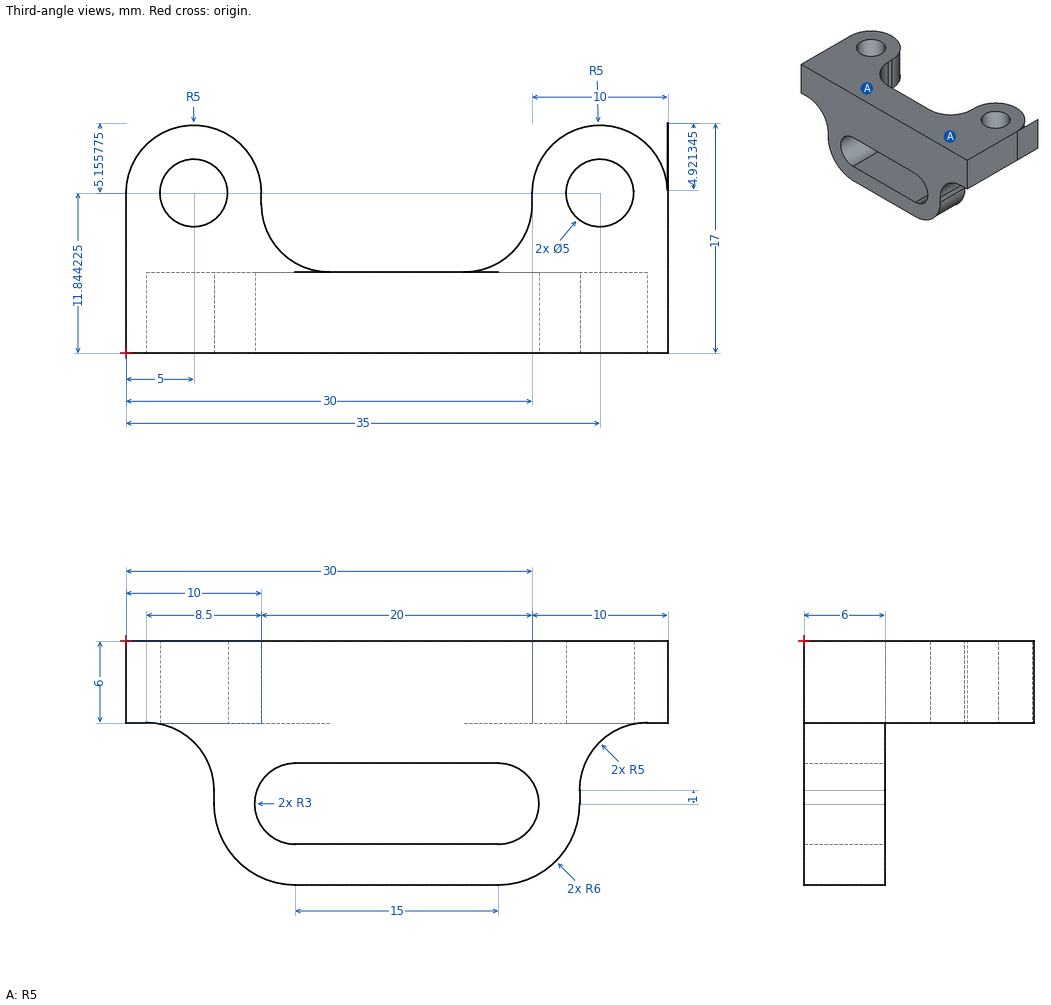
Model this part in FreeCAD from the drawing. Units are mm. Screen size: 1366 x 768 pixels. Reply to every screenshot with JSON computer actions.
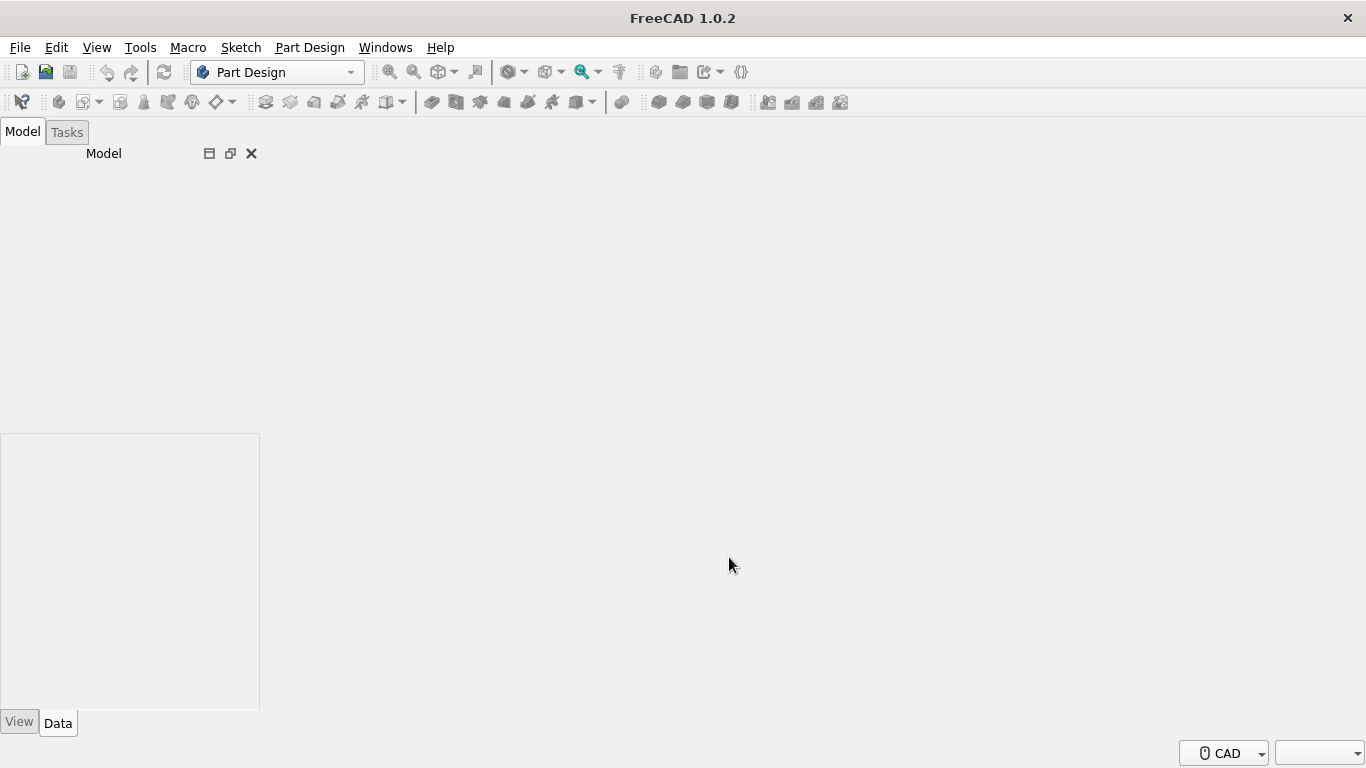
{"action": "key", "text": "ctrl+n"}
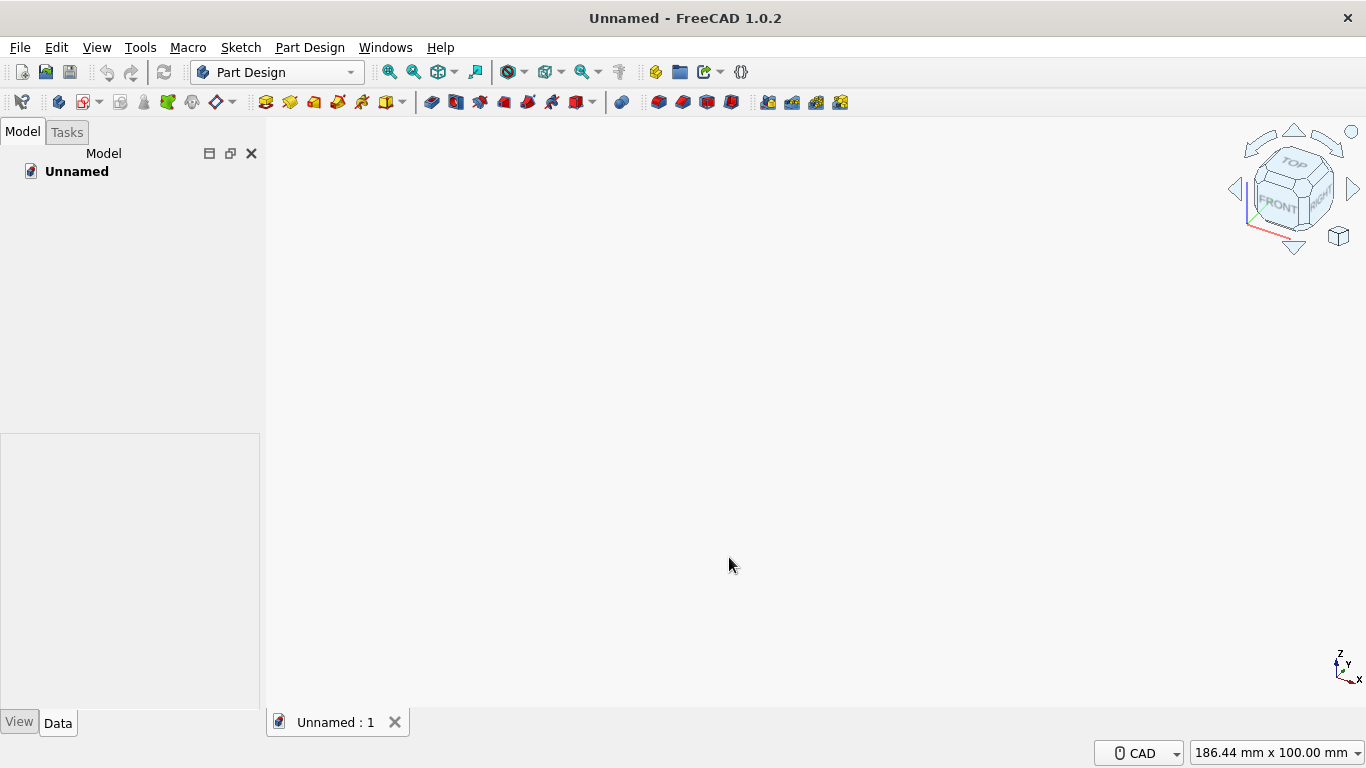
{"action": "left_click", "coordinate": [84, 102]}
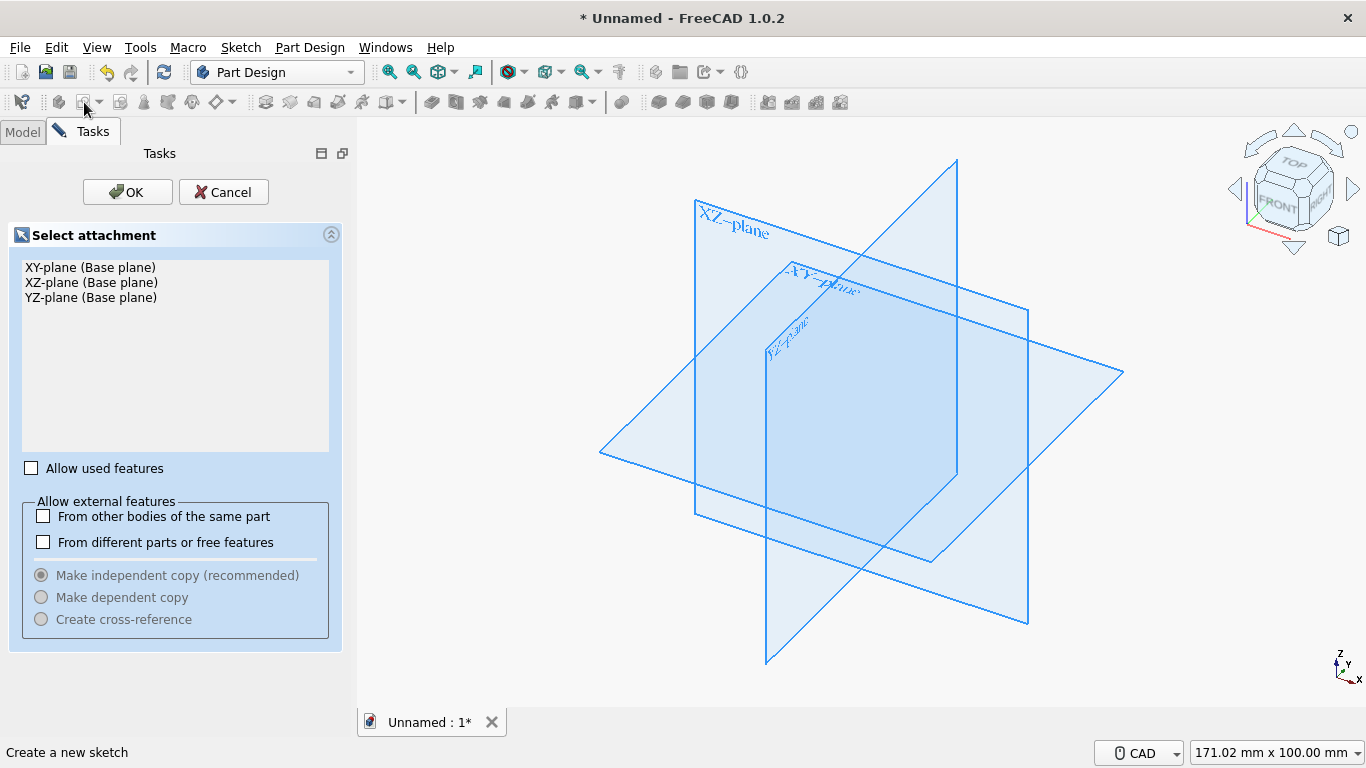
{"action": "left_click", "coordinate": [82, 282]}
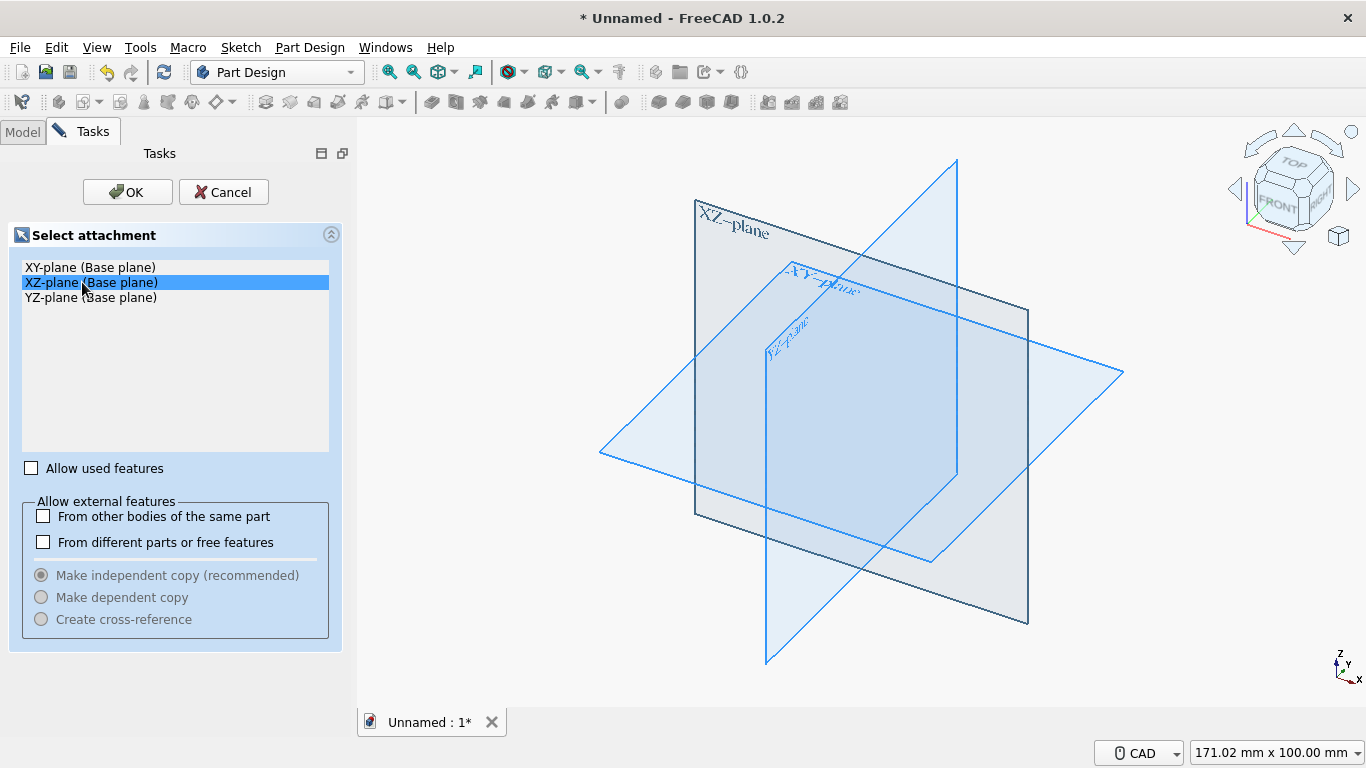
{"action": "left_click", "coordinate": [128, 192]}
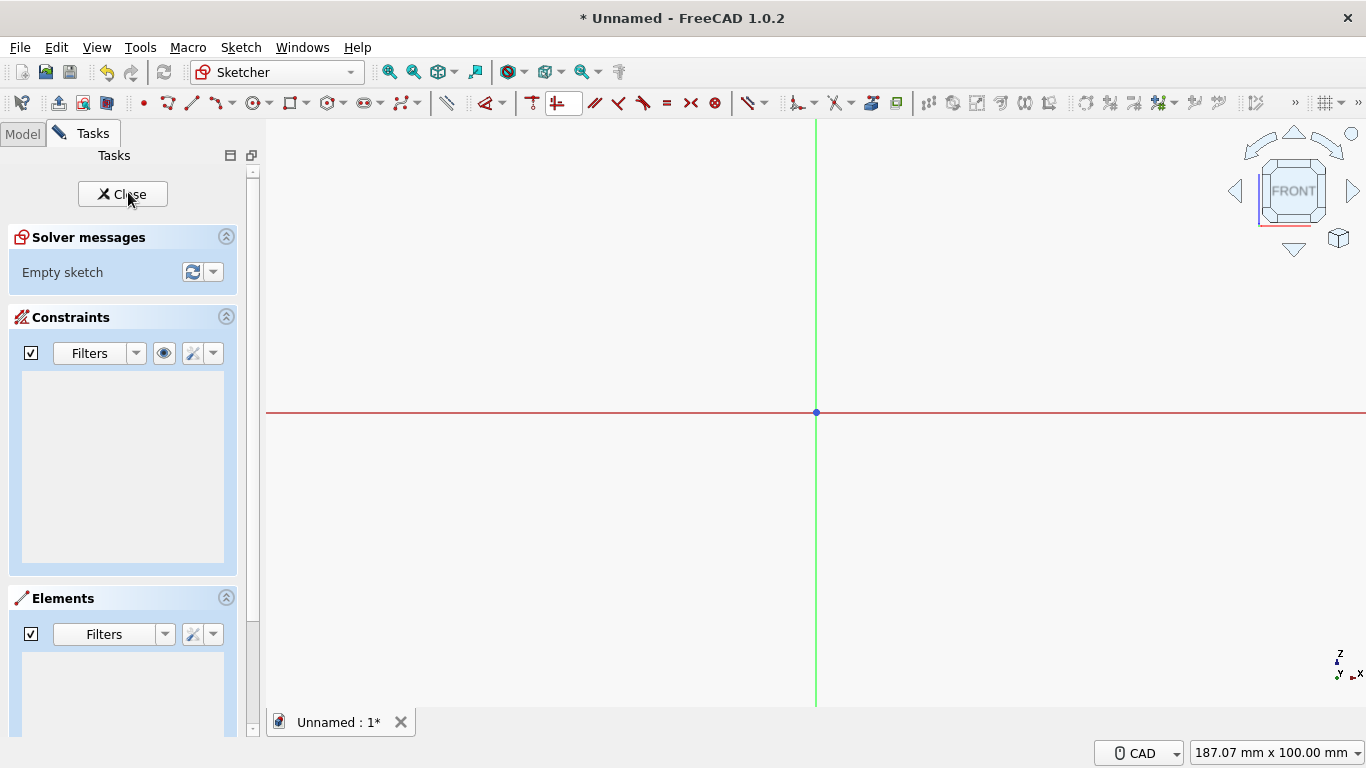
{"action": "scroll", "coordinate": [1035, 497], "scroll_direction": "up", "scroll_amount": 5}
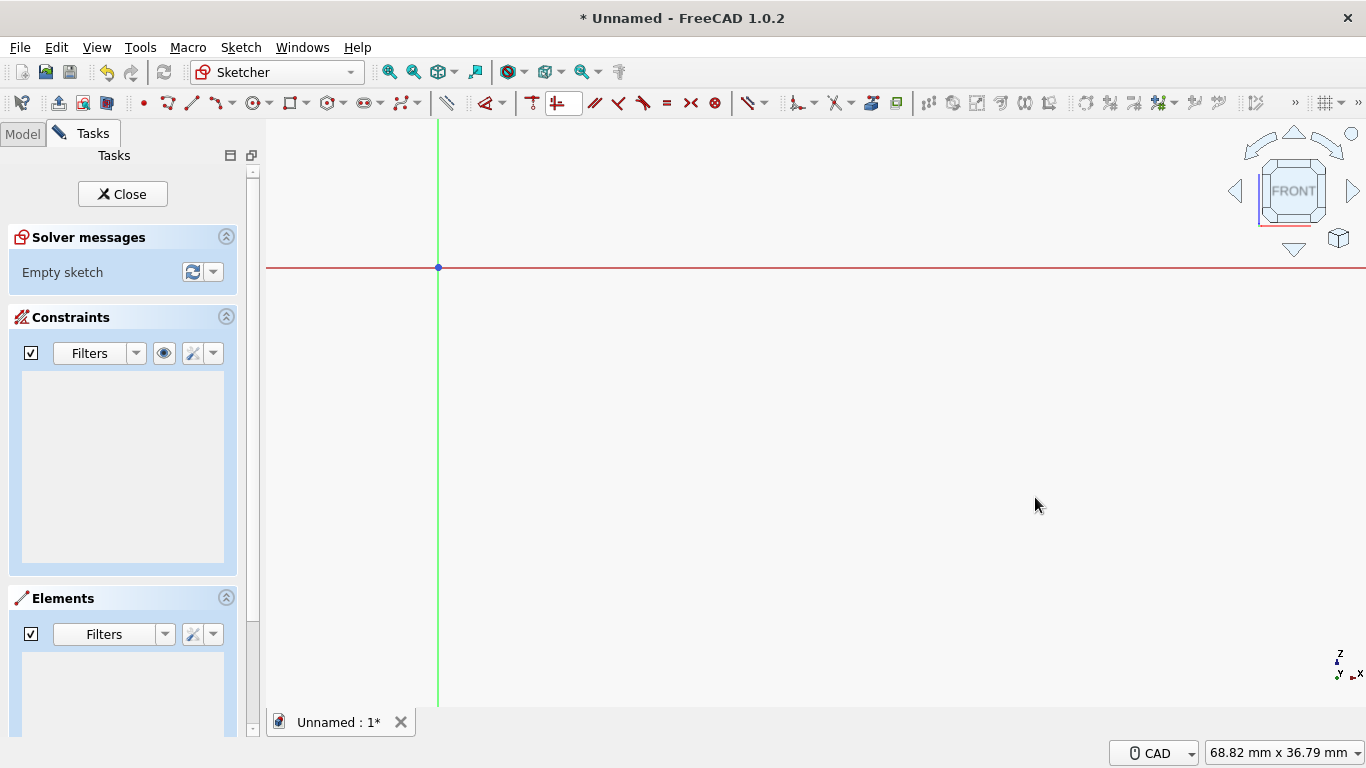
{"action": "left_click", "coordinate": [192, 104]}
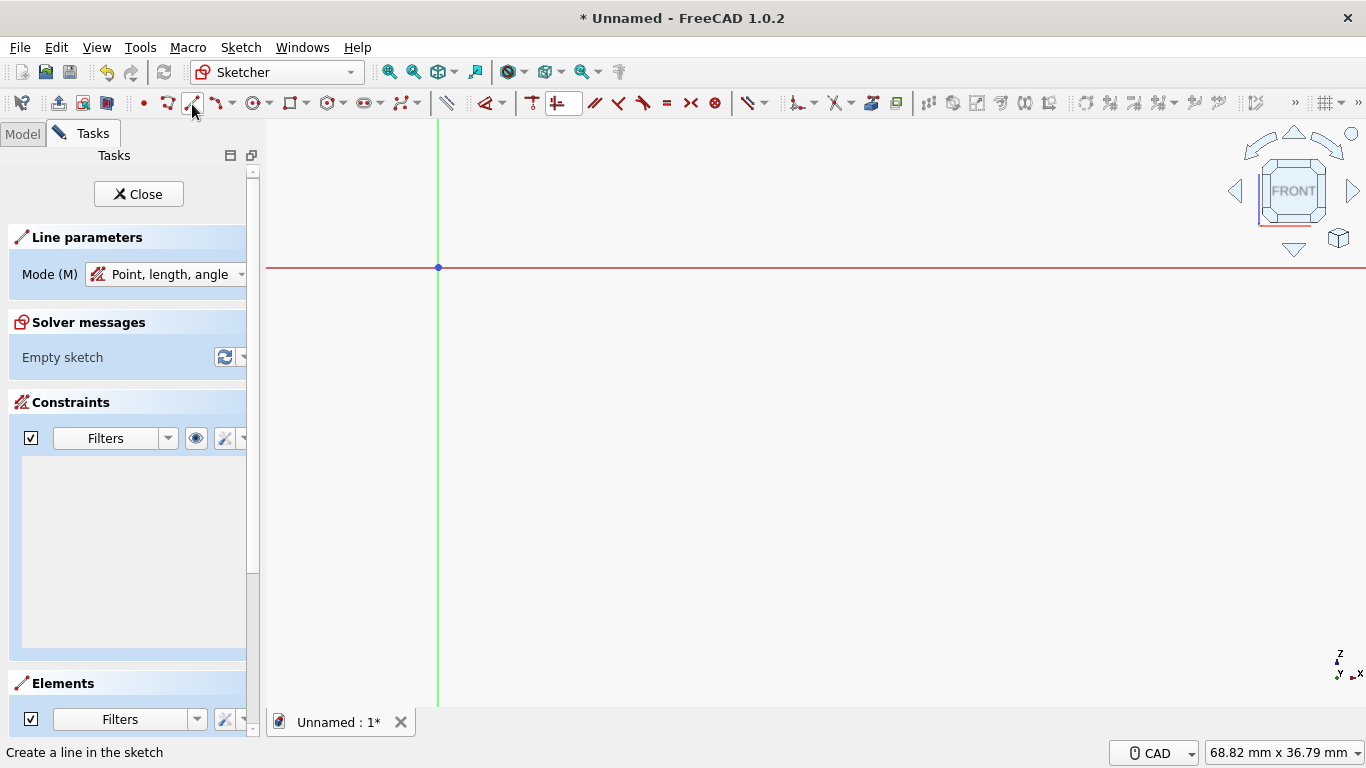
{"action": "left_click", "coordinate": [974, 443]}
{"action": "left_click", "coordinate": [974, 459]}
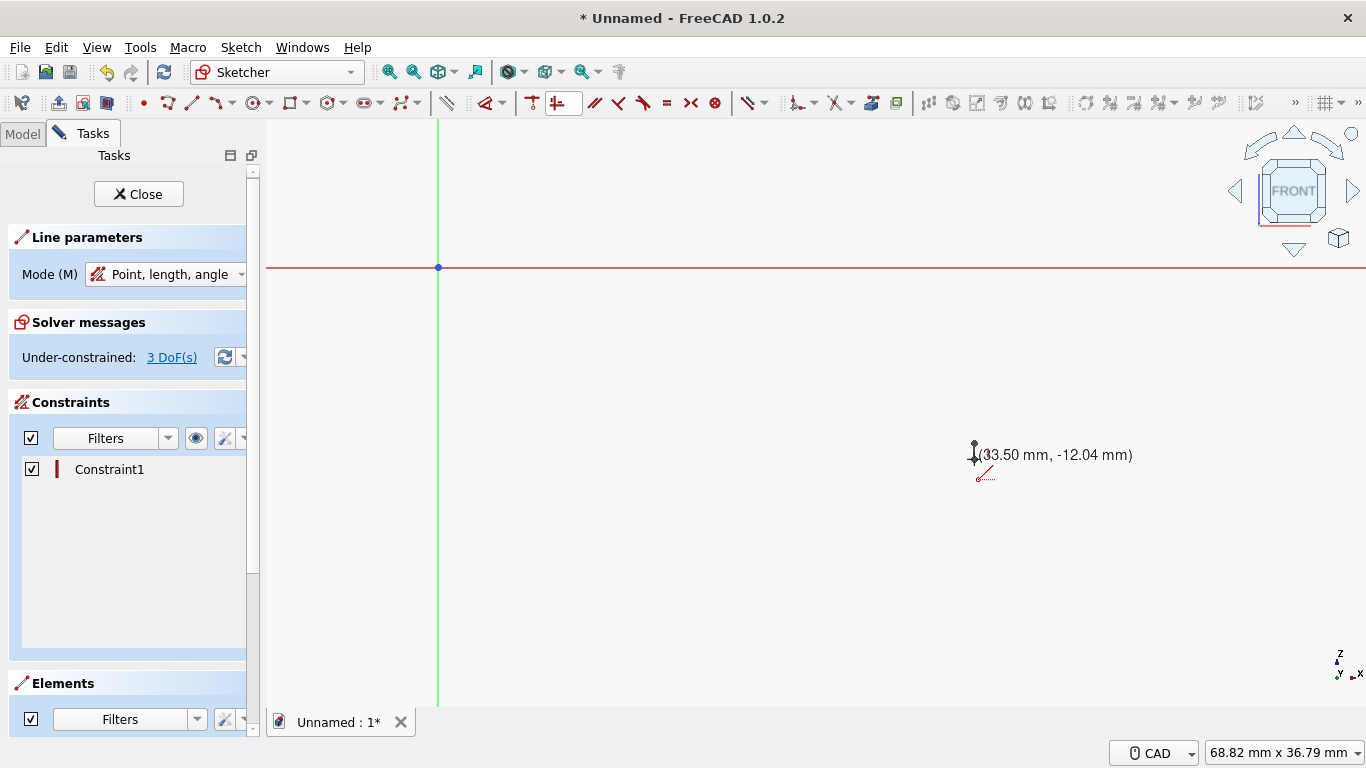
{"action": "left_click", "coordinate": [878, 555]}
{"action": "left_click", "coordinate": [638, 555]}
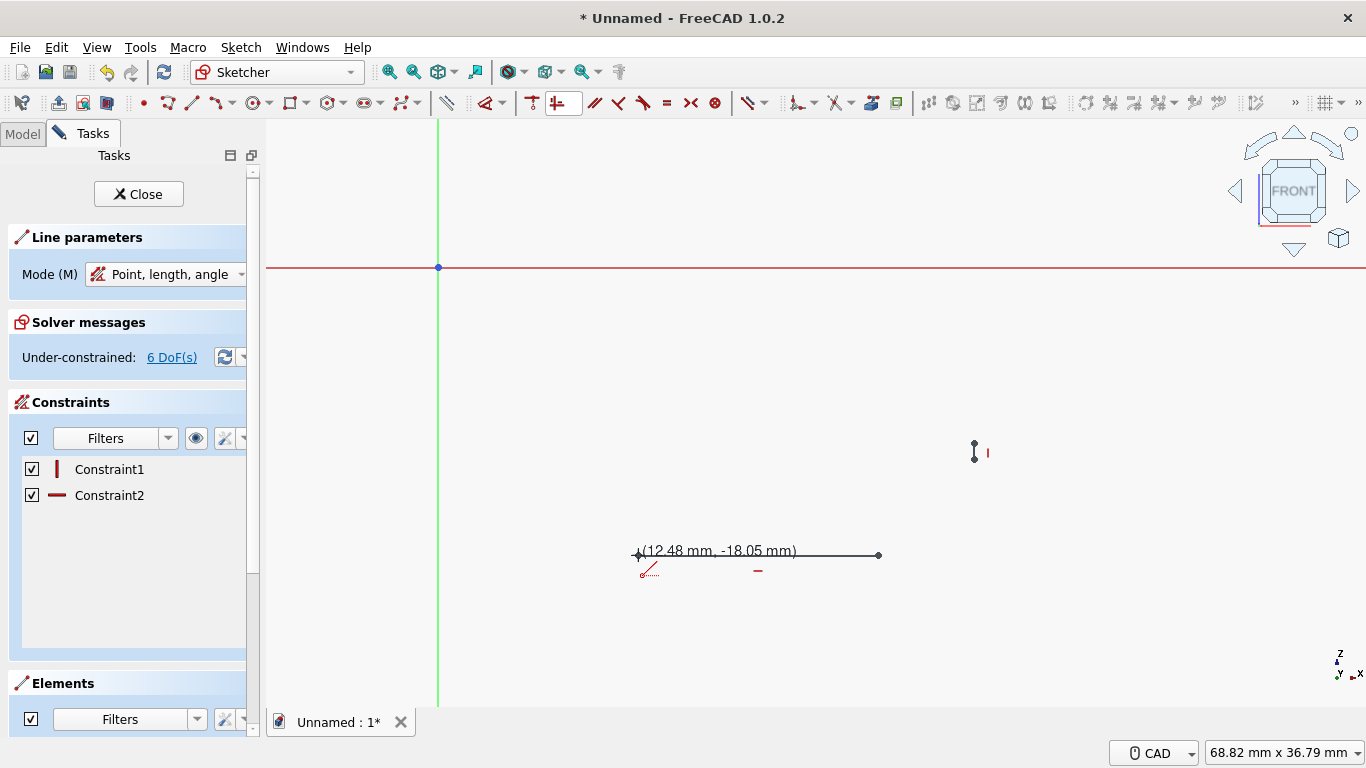
{"action": "left_click", "coordinate": [542, 459]}
{"action": "left_click", "coordinate": [542, 443]}